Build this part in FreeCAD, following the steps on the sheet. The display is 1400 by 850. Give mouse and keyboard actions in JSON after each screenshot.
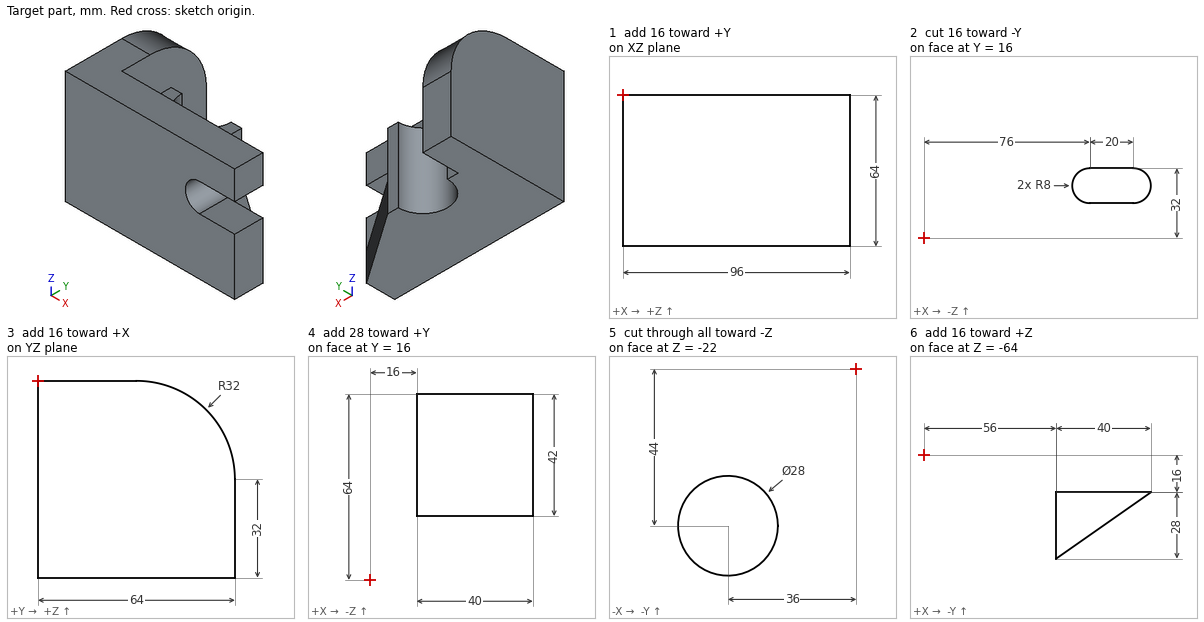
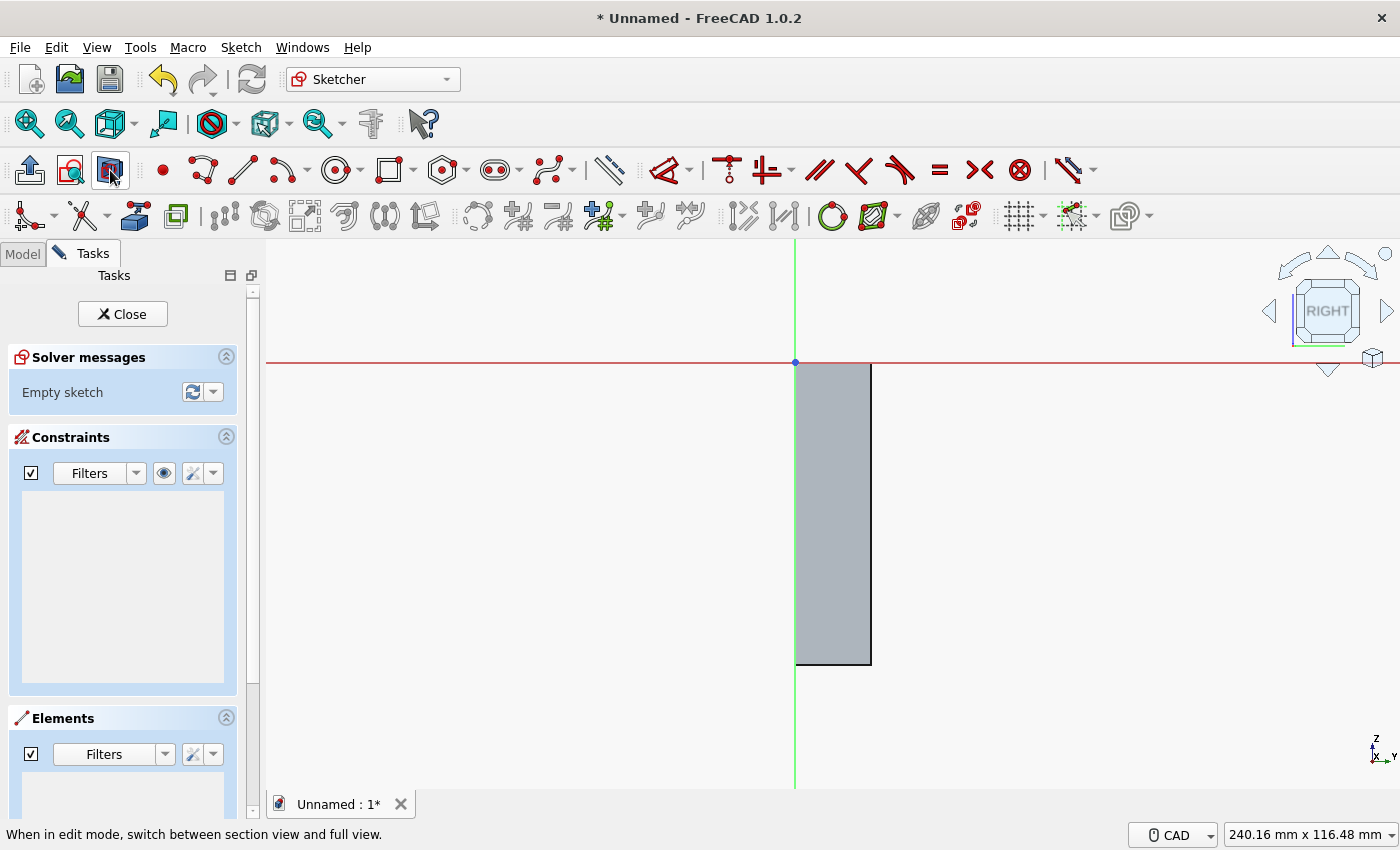
{"action": "left_click", "coordinate": [204, 170]}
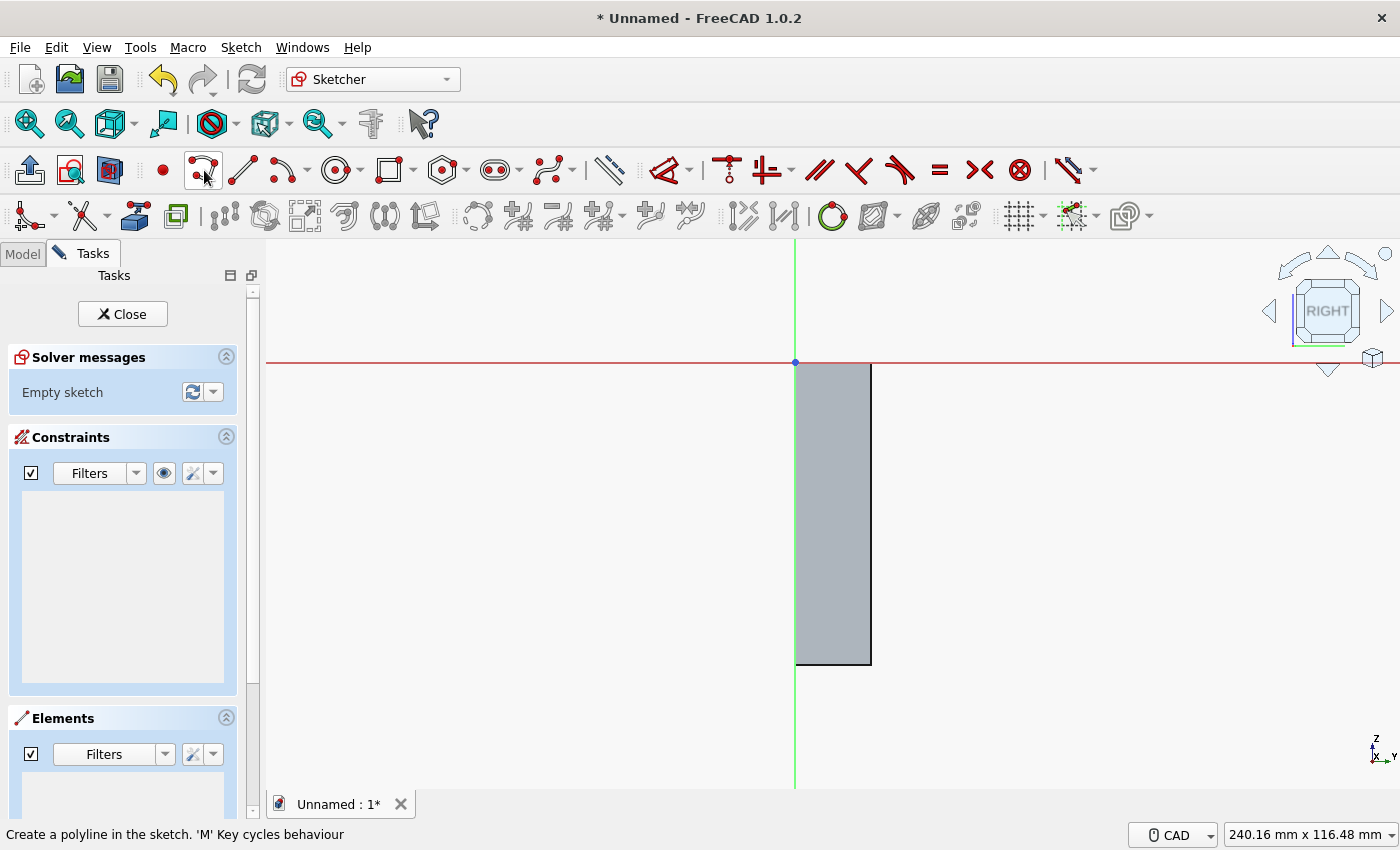
{"action": "left_click", "coordinate": [1097, 514]}
{"action": "left_click", "coordinate": [1097, 665]}
{"action": "left_click", "coordinate": [795, 665]}
{"action": "left_click", "coordinate": [795, 363]}
{"action": "left_click", "coordinate": [946, 372]}
{"action": "right_click", "coordinate": [946, 372]}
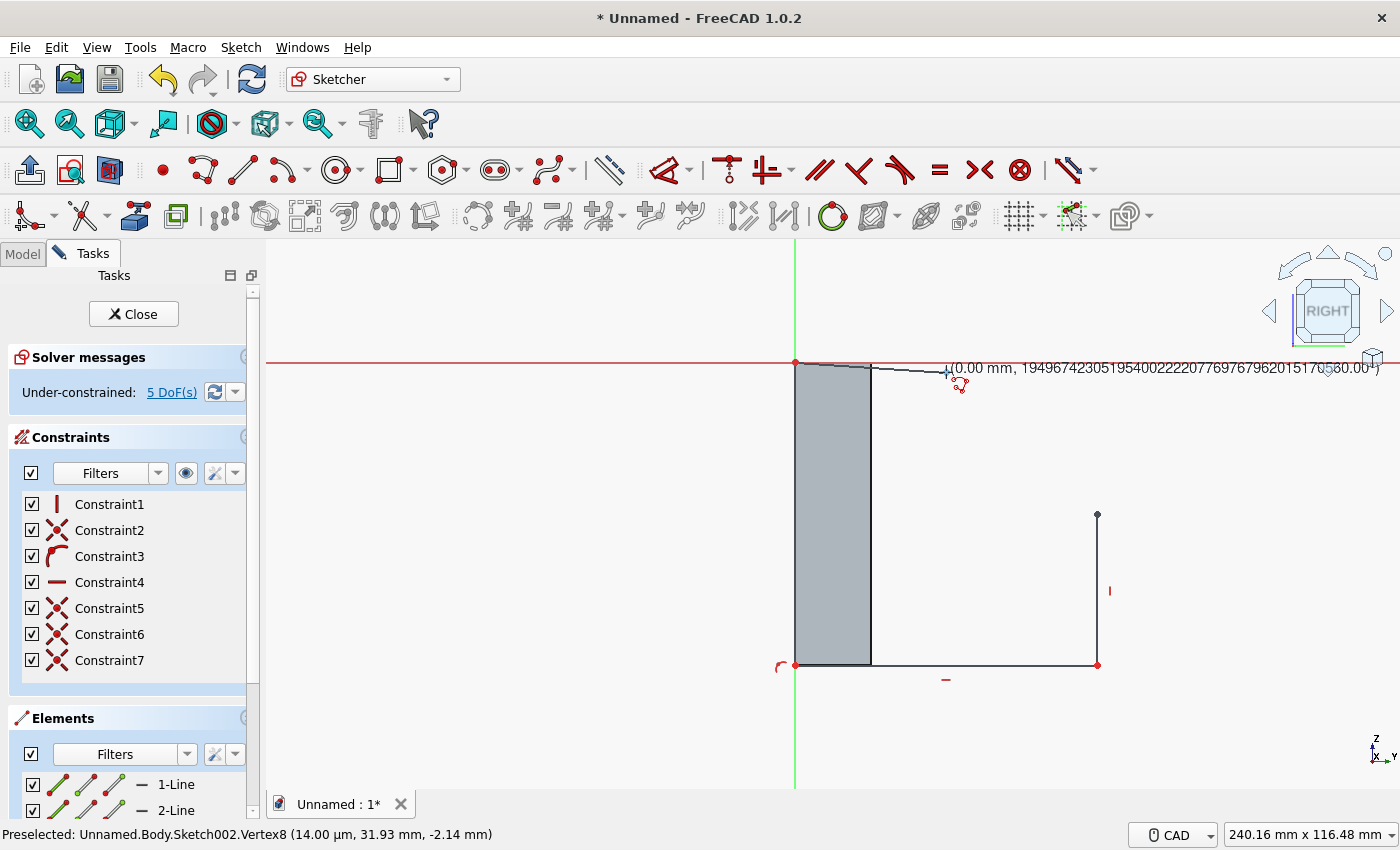
{"action": "left_click", "coordinate": [310, 170]}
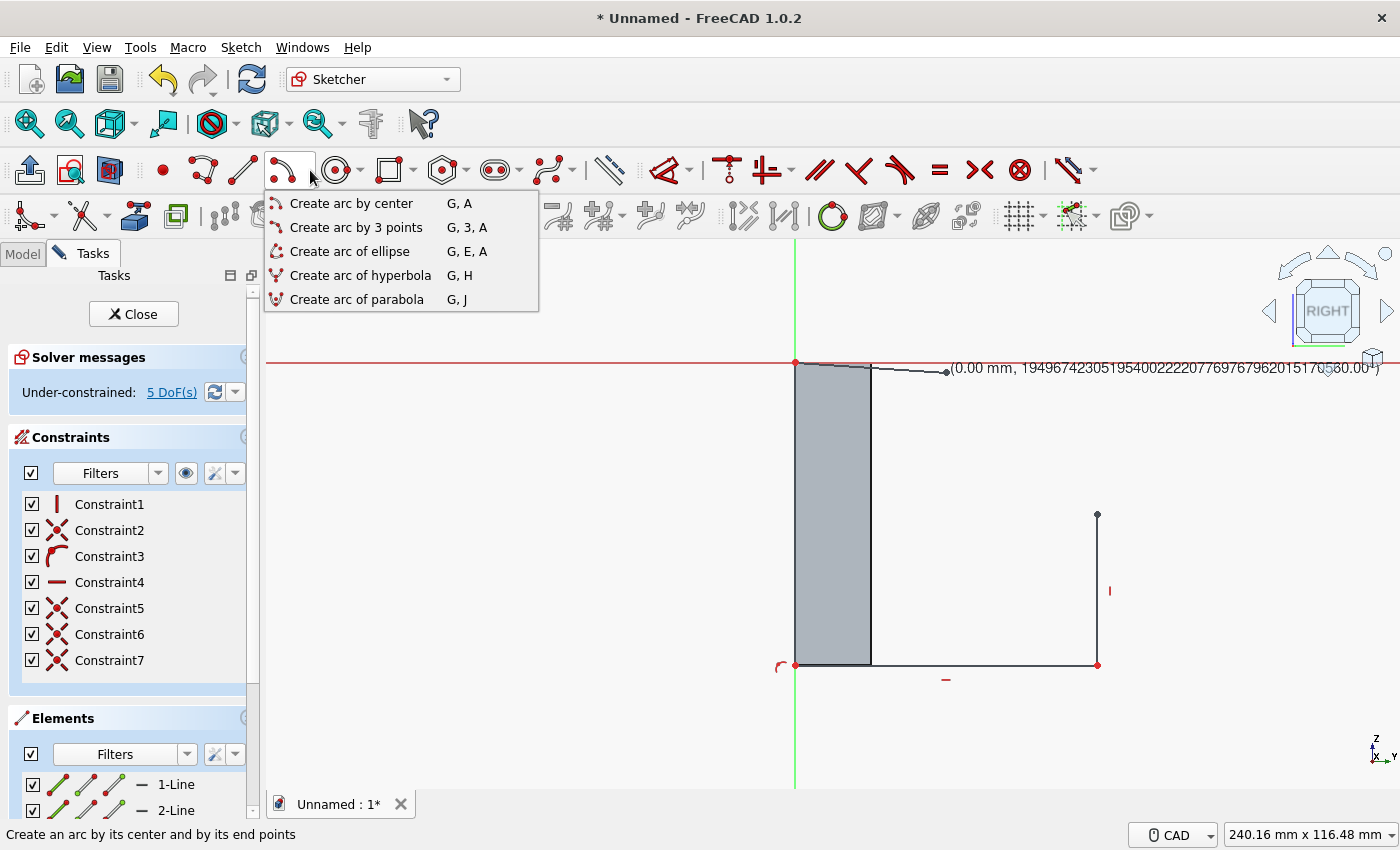
{"action": "left_click", "coordinate": [402, 227]}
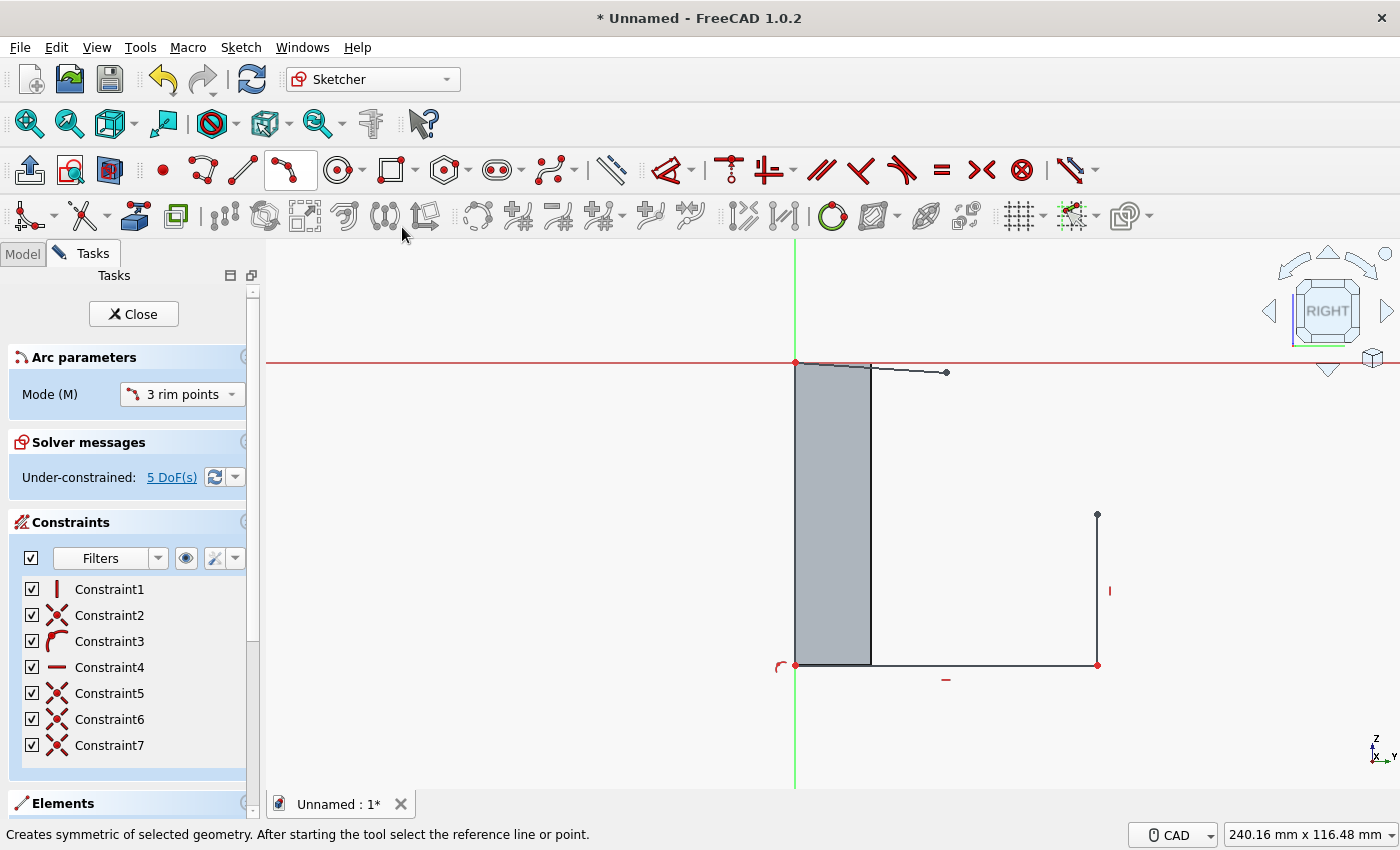
{"action": "left_click", "coordinate": [946, 373]}
{"action": "left_click", "coordinate": [1097, 515]}
{"action": "left_click", "coordinate": [1053, 407]}
{"action": "key", "text": "Escape"}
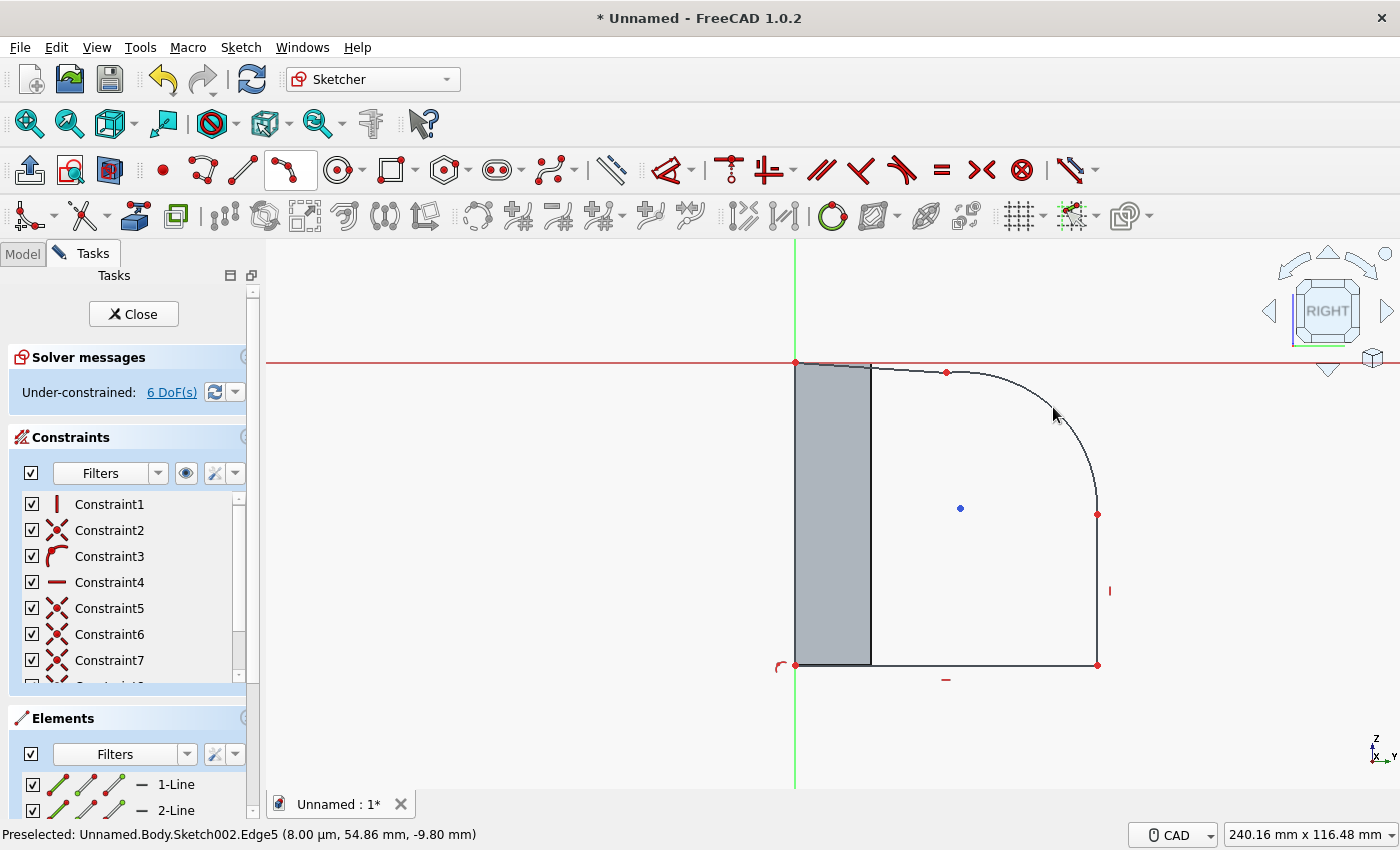
{"action": "left_click", "coordinate": [1097, 560]}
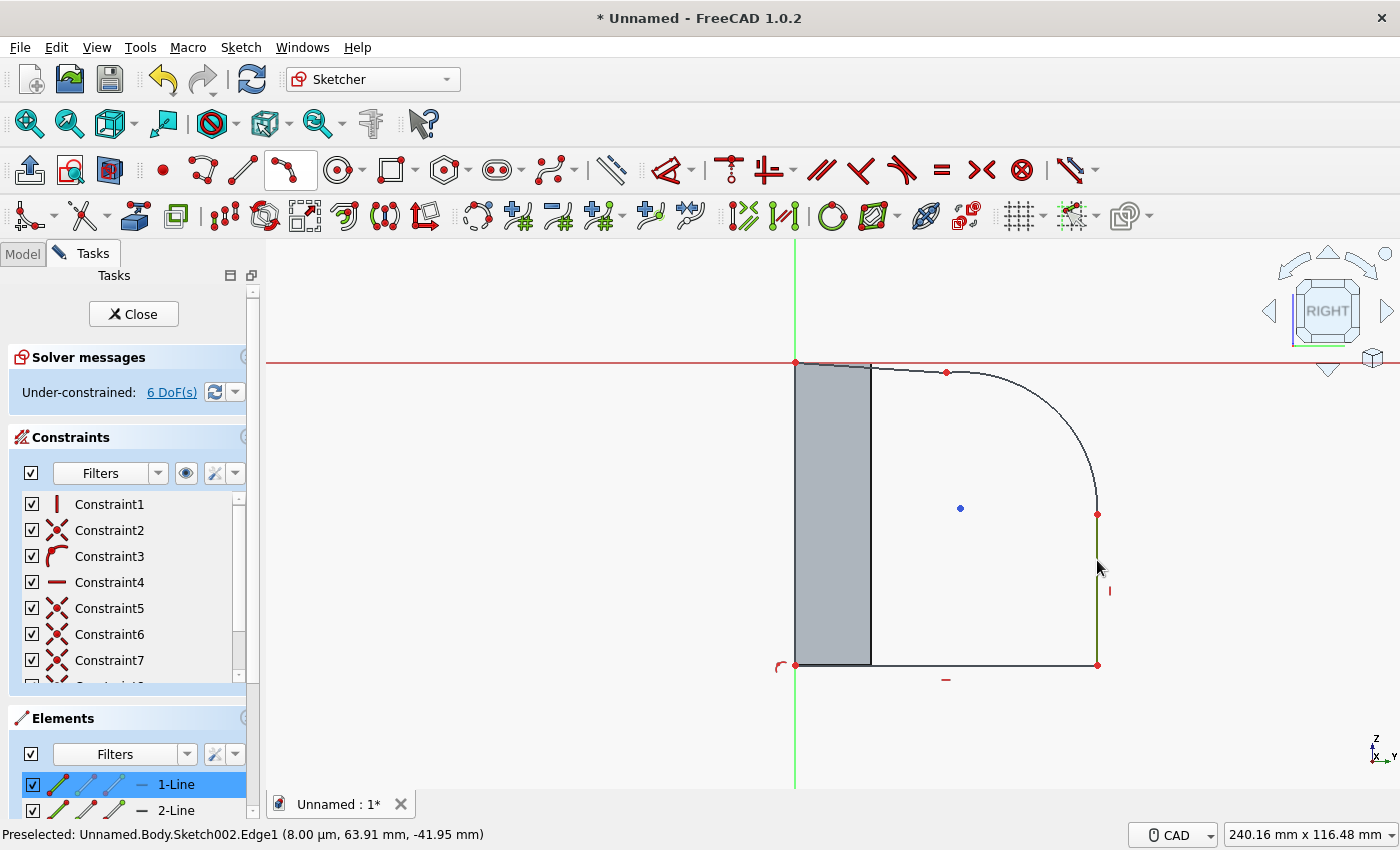
{"action": "left_click", "coordinate": [1082, 447]}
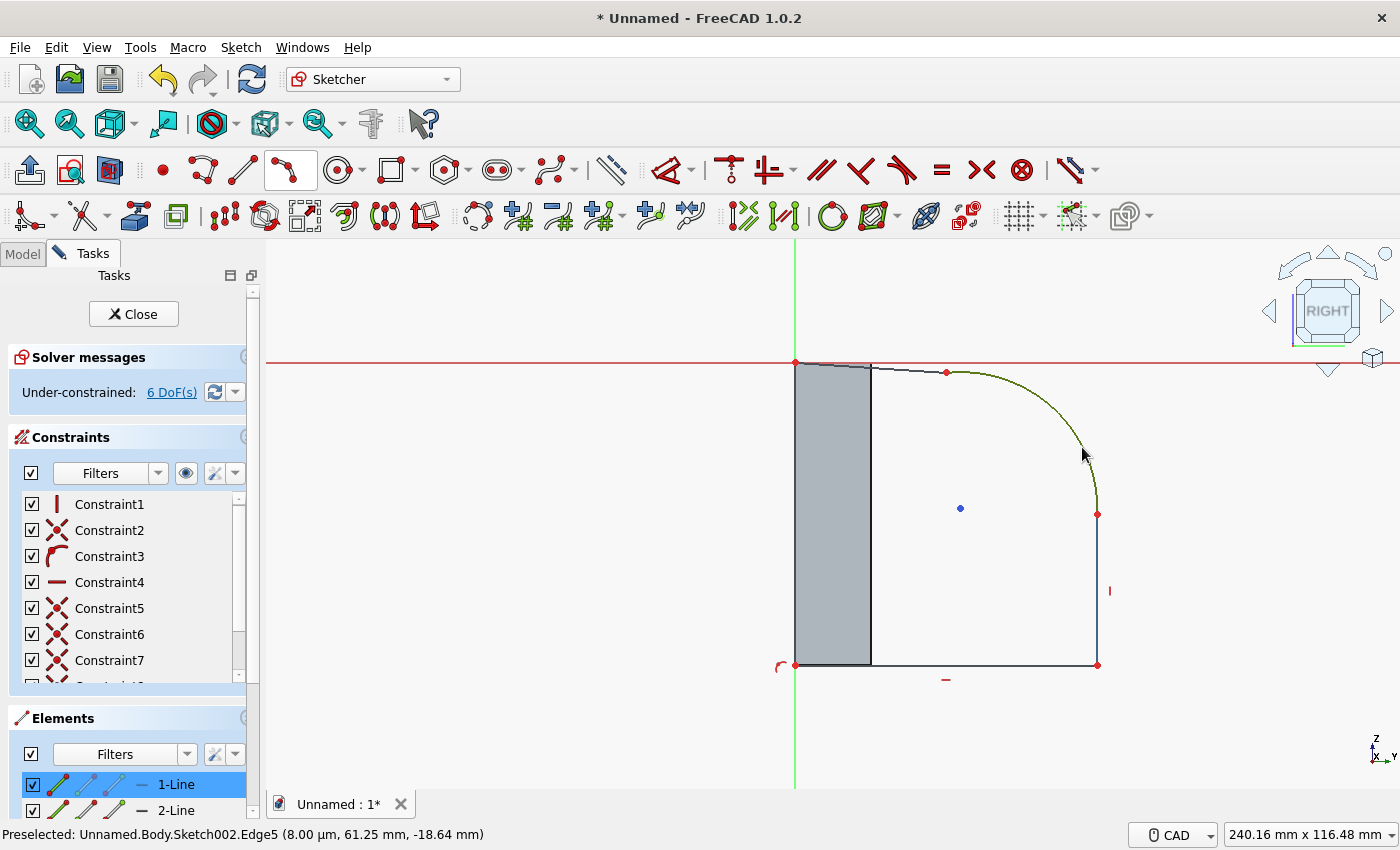
{"action": "left_click", "coordinate": [902, 170]}